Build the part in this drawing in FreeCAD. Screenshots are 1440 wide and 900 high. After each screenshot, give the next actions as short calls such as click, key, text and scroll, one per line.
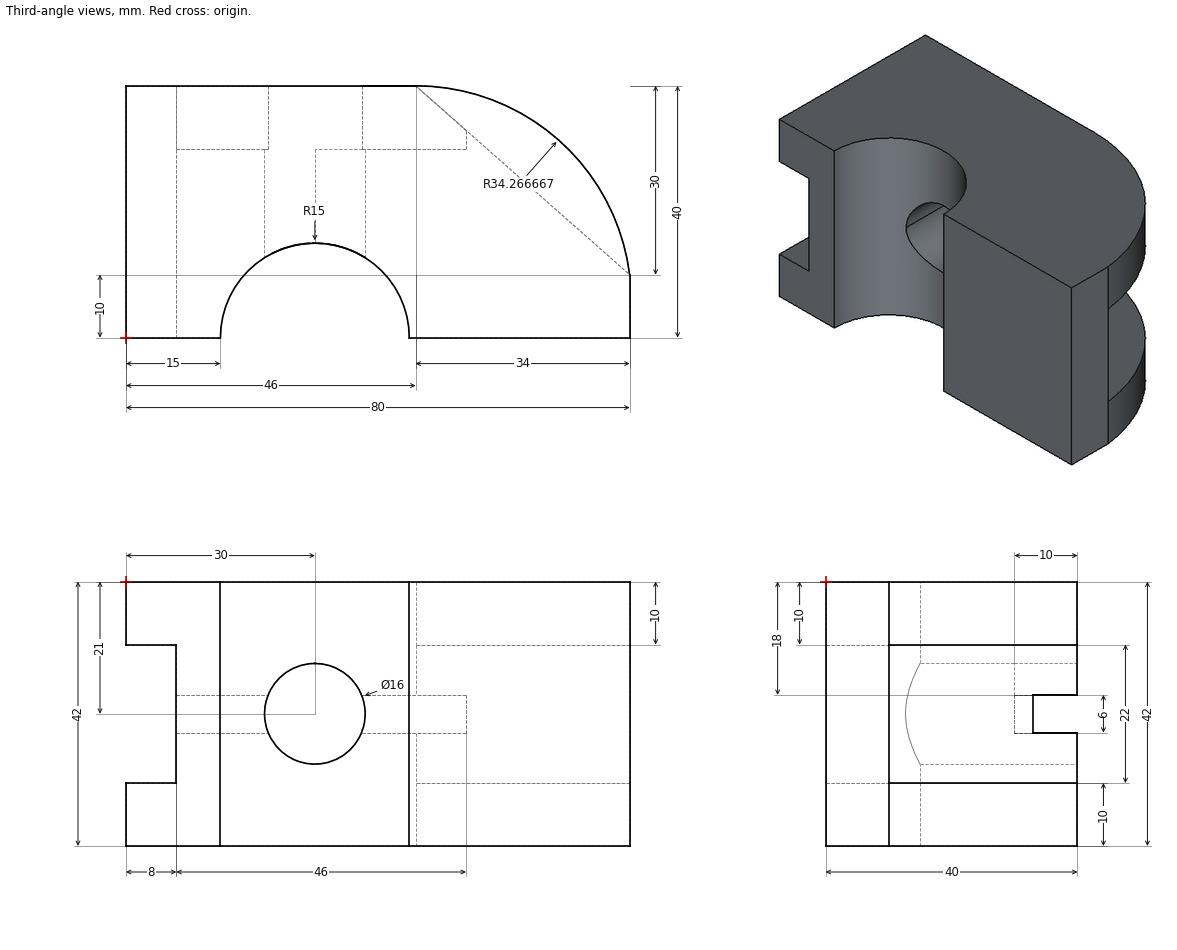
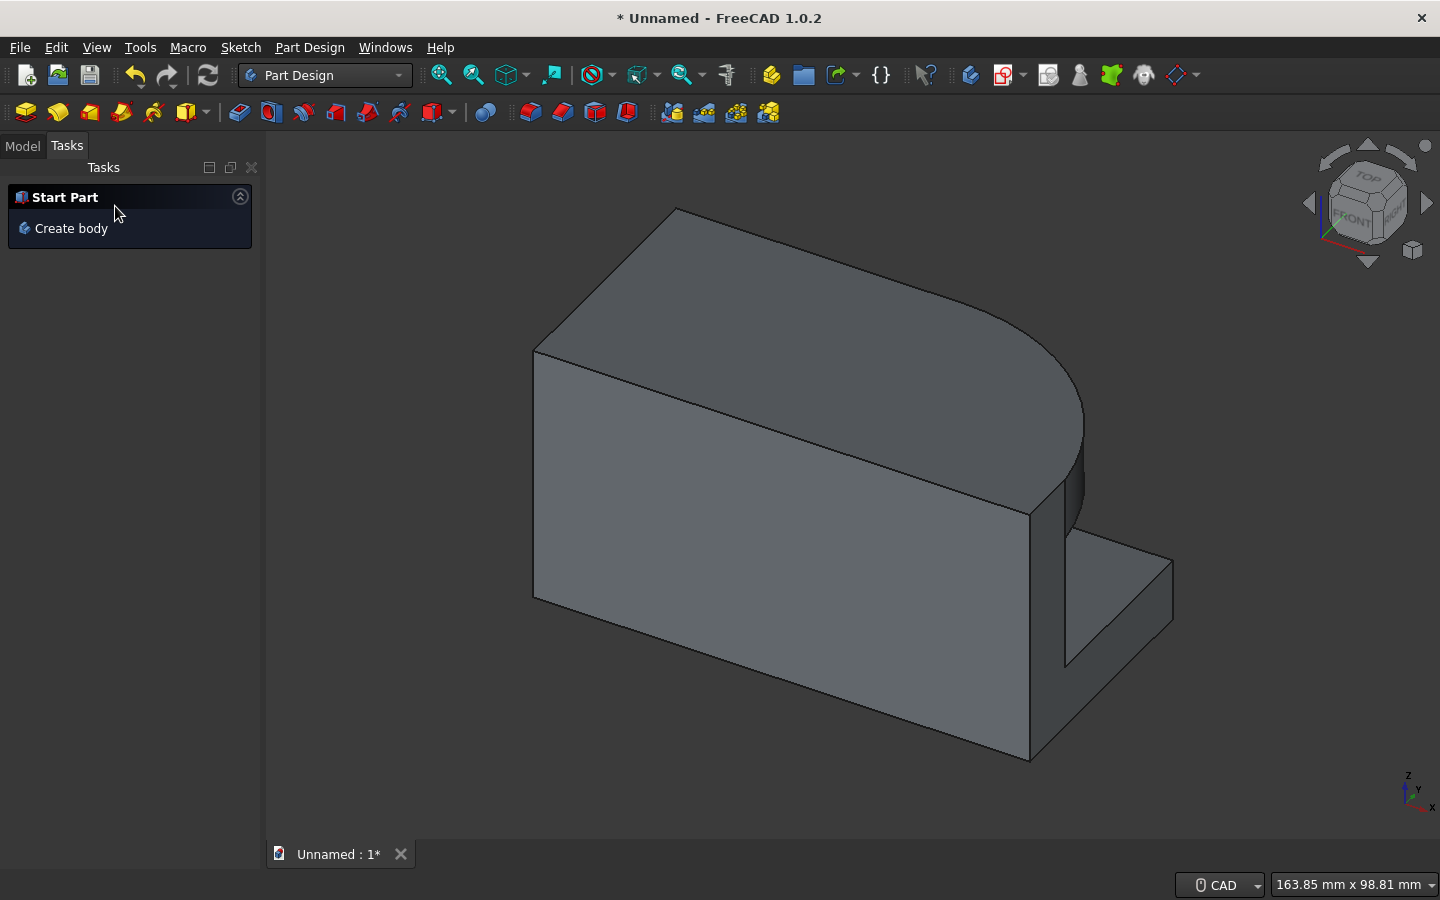
click(1089, 583)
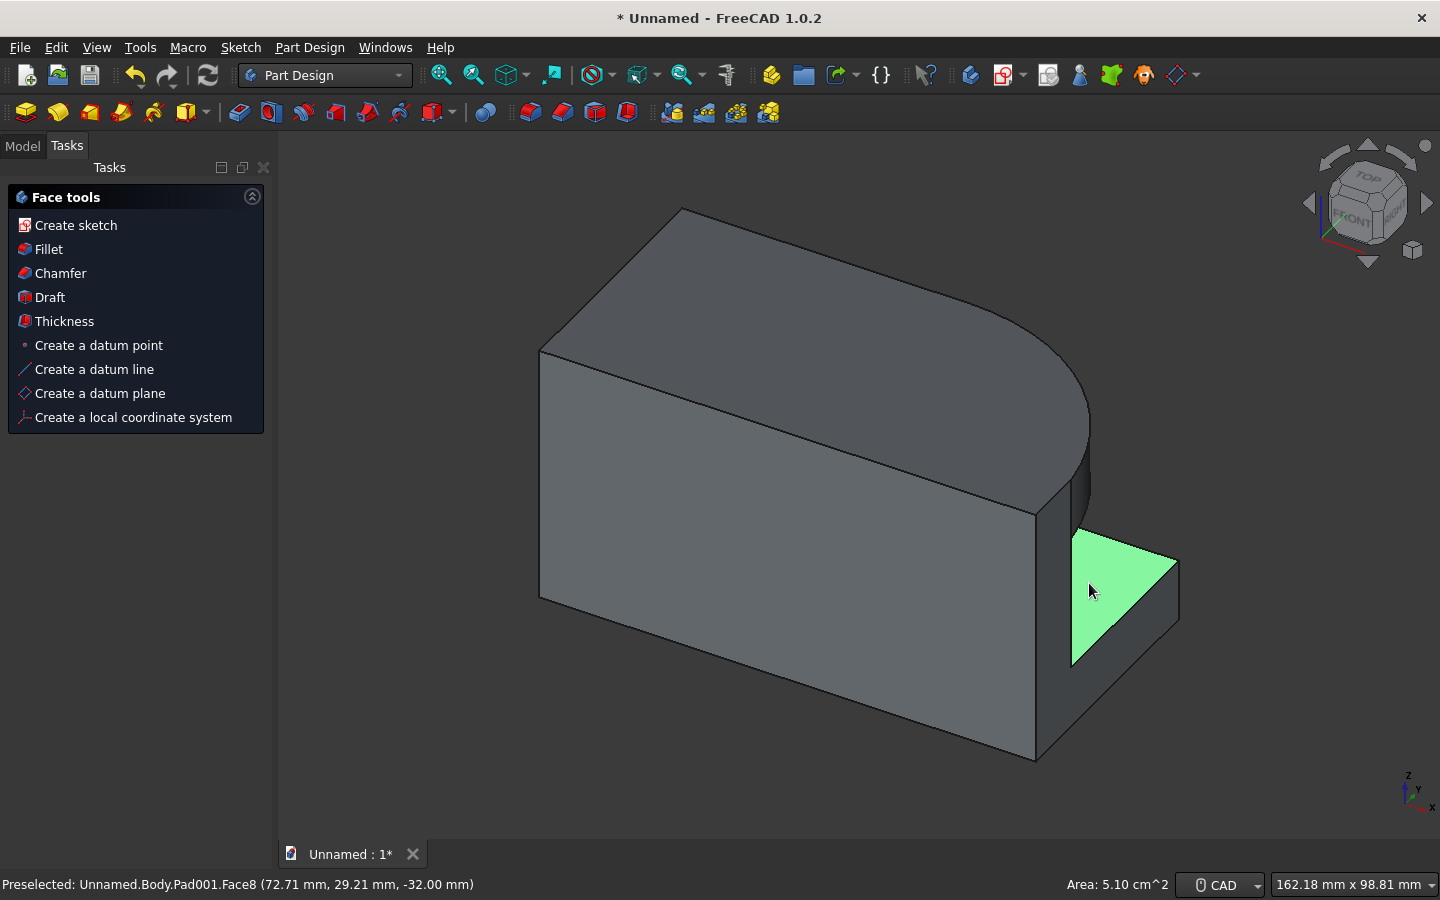
click(1004, 76)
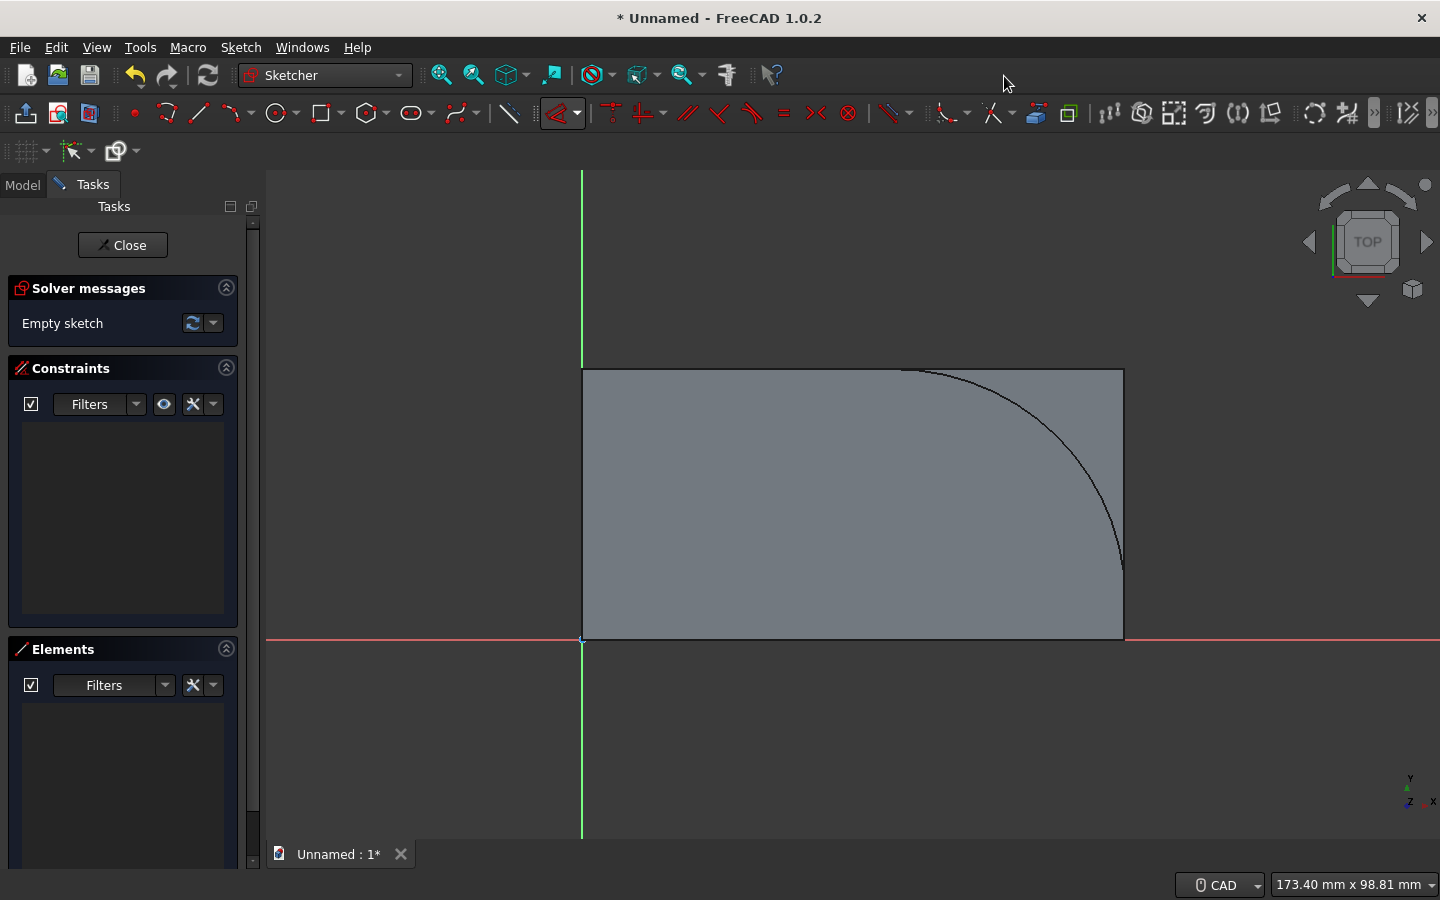
click(90, 114)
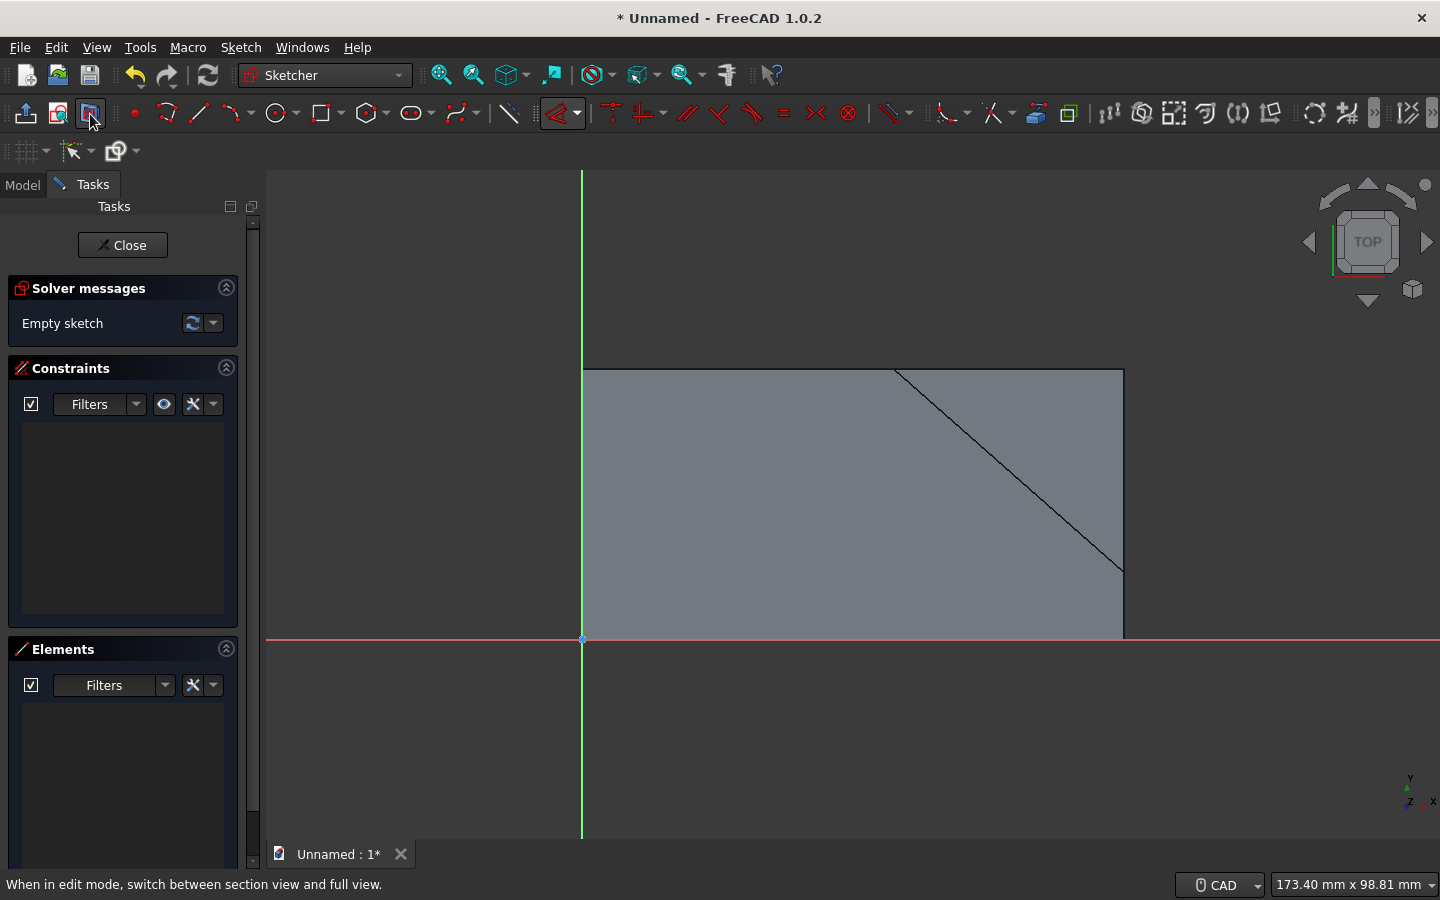
click(168, 114)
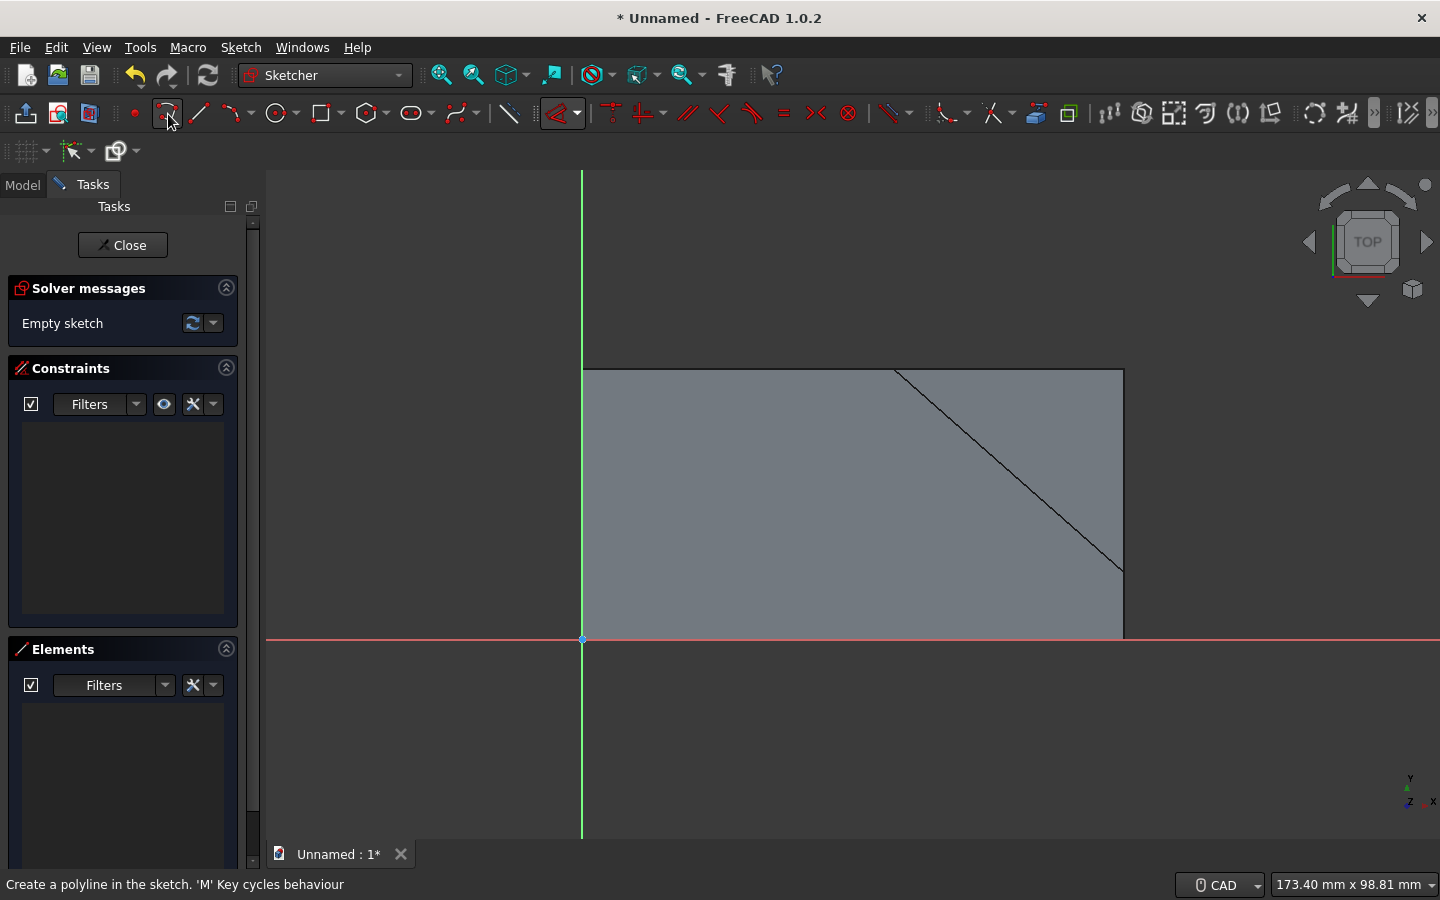
click(1124, 572)
click(1124, 369)
click(894, 369)
right_click(894, 369)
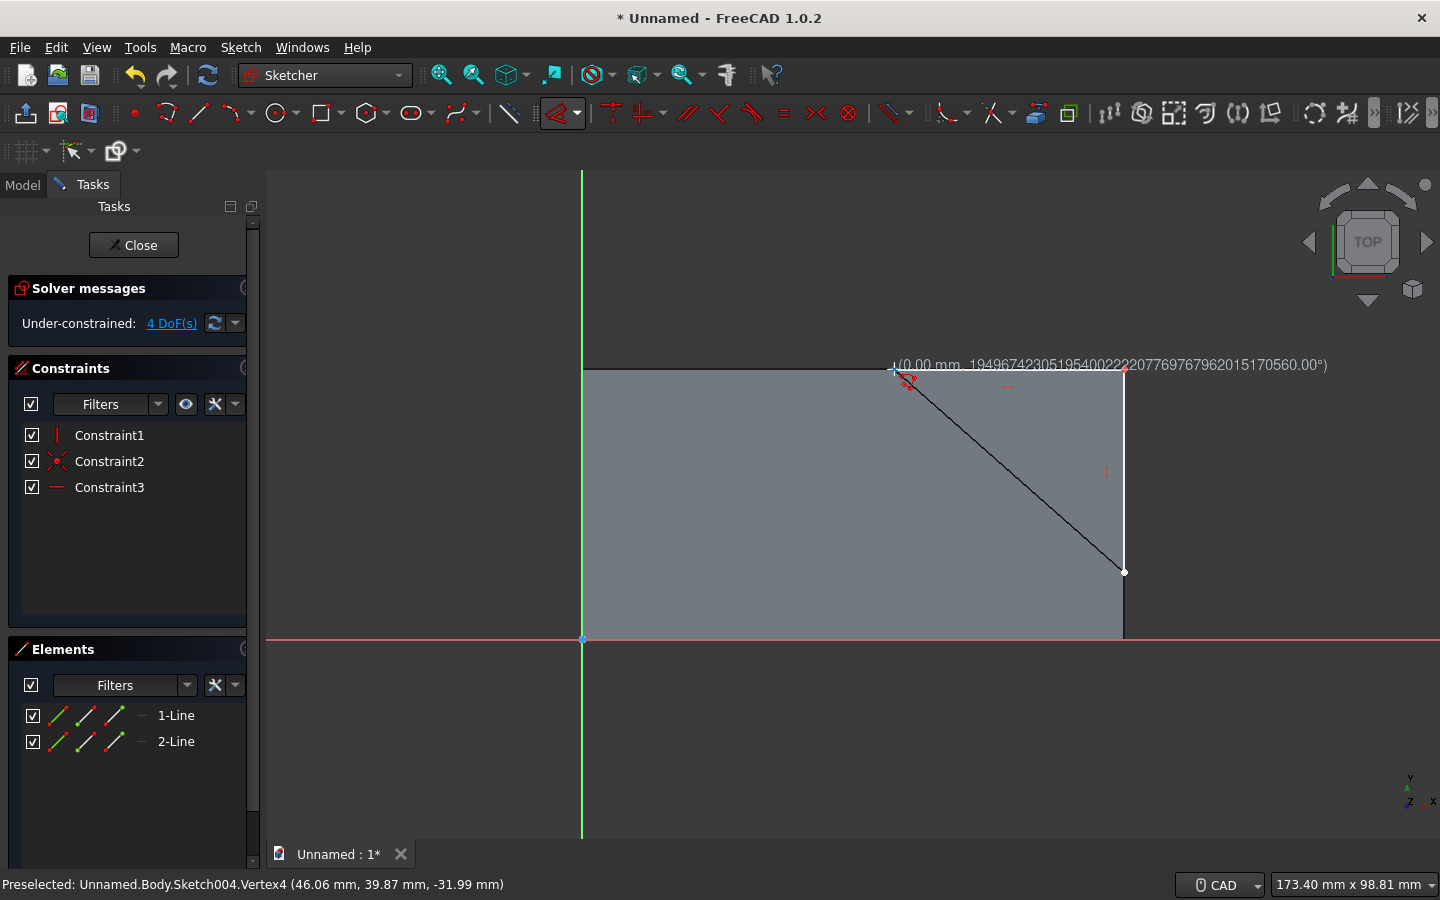
click(232, 114)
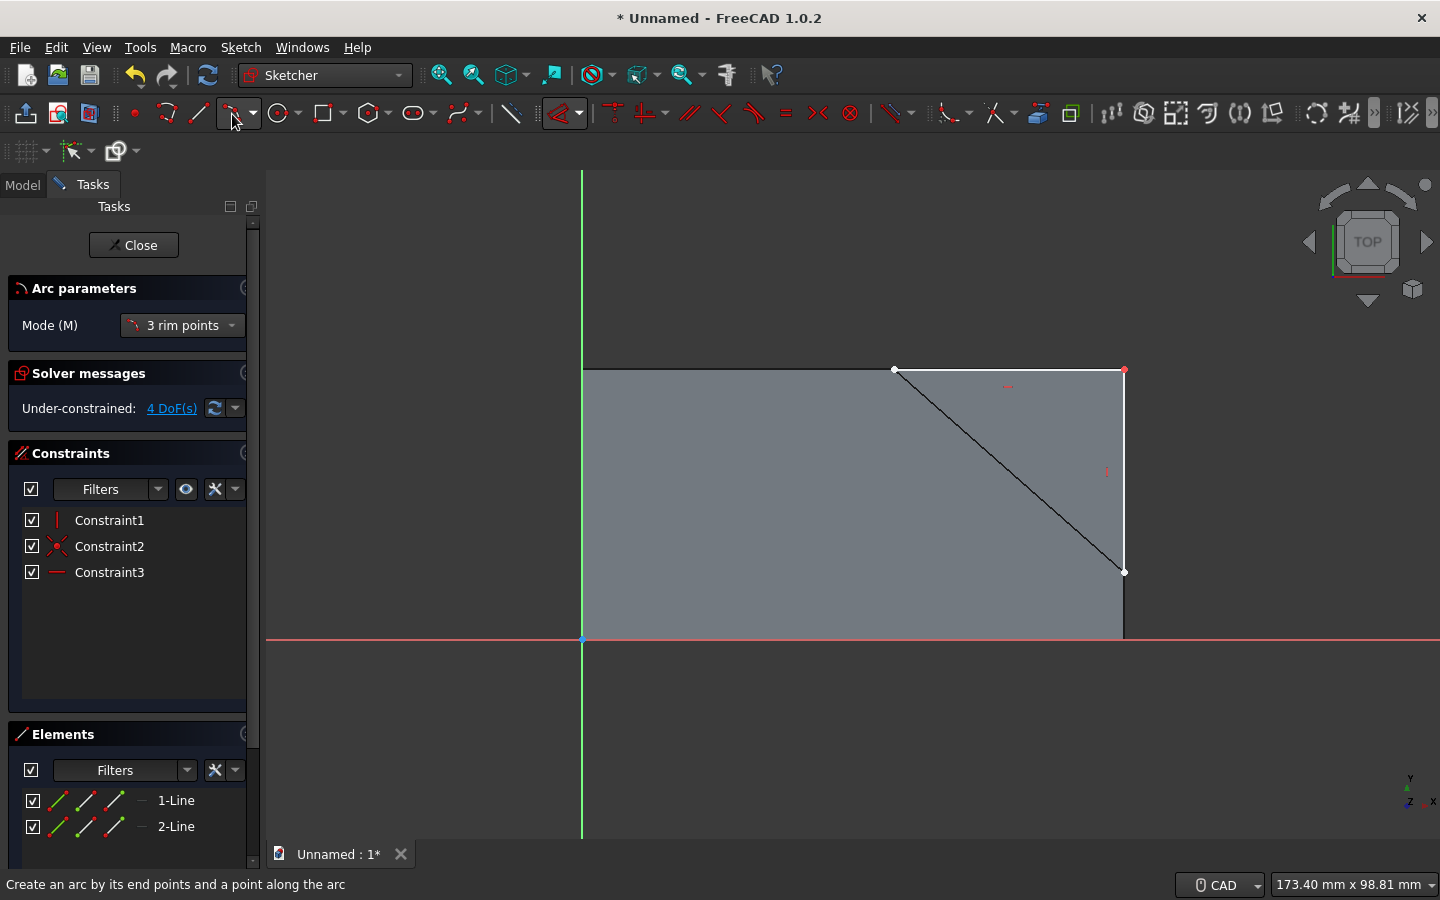
click(894, 370)
click(1124, 573)
click(1047, 427)
key(Escape)